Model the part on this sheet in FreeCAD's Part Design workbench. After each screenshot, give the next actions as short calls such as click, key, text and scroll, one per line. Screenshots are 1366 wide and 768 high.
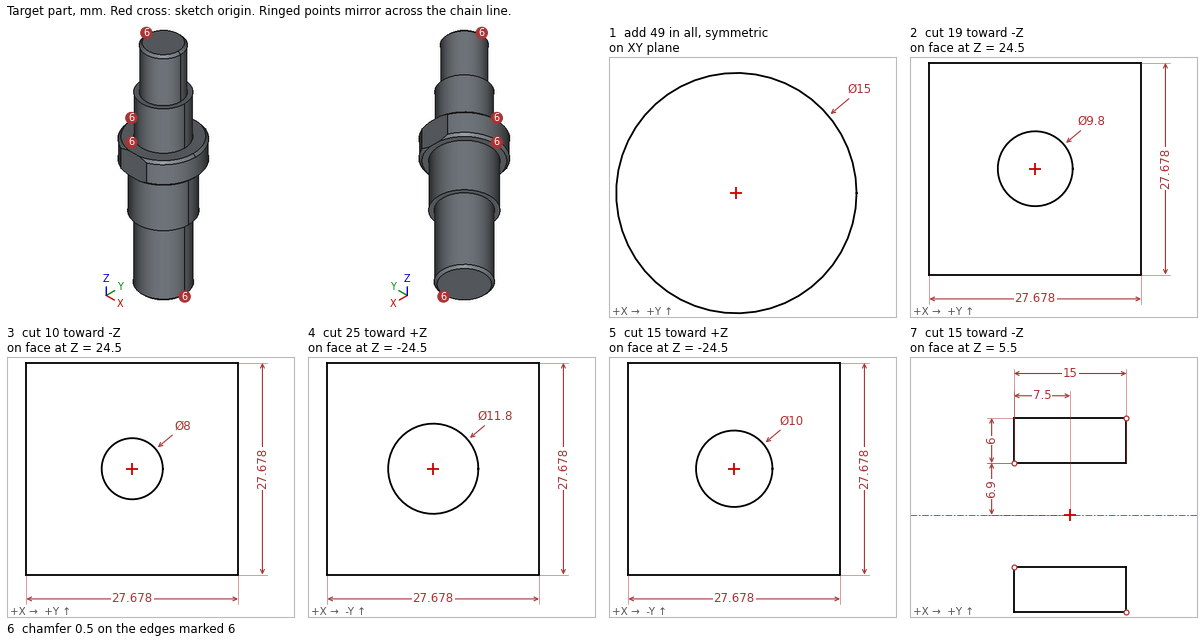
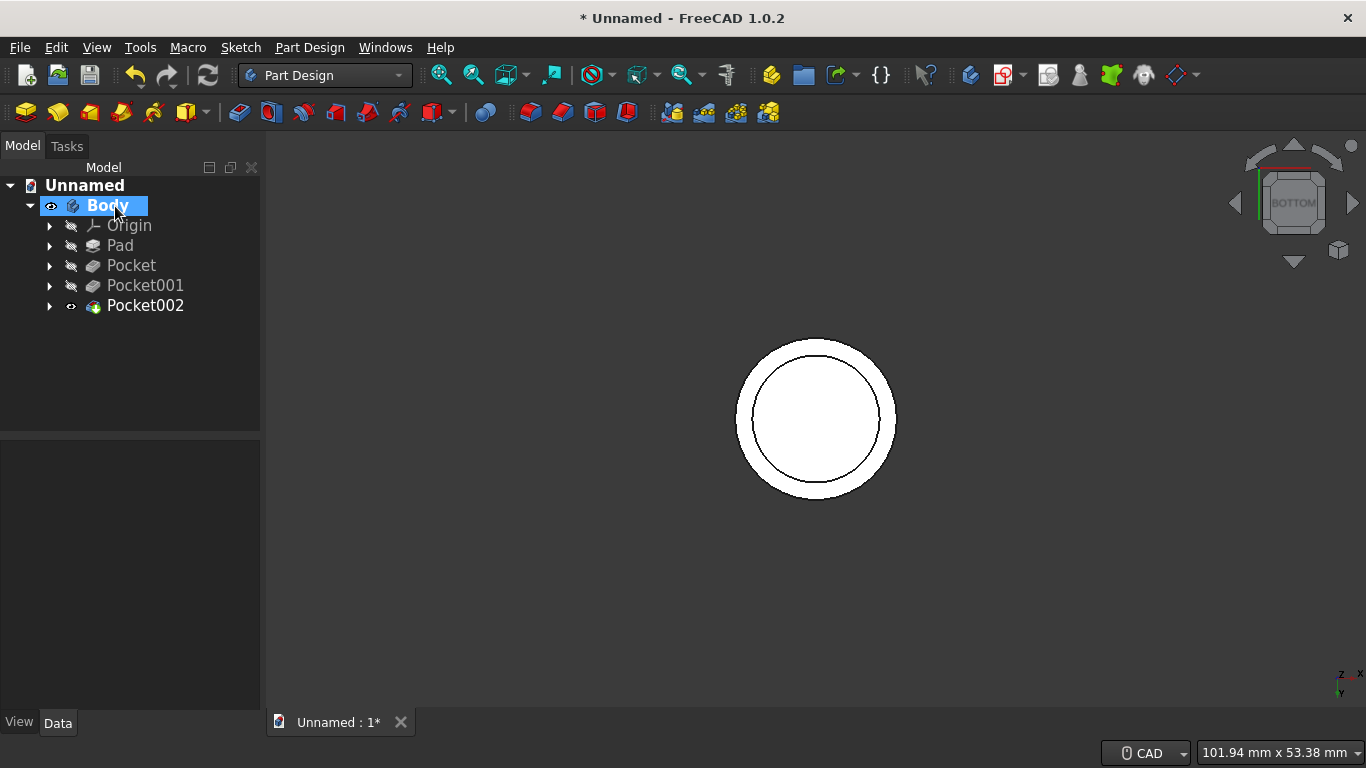
click(442, 76)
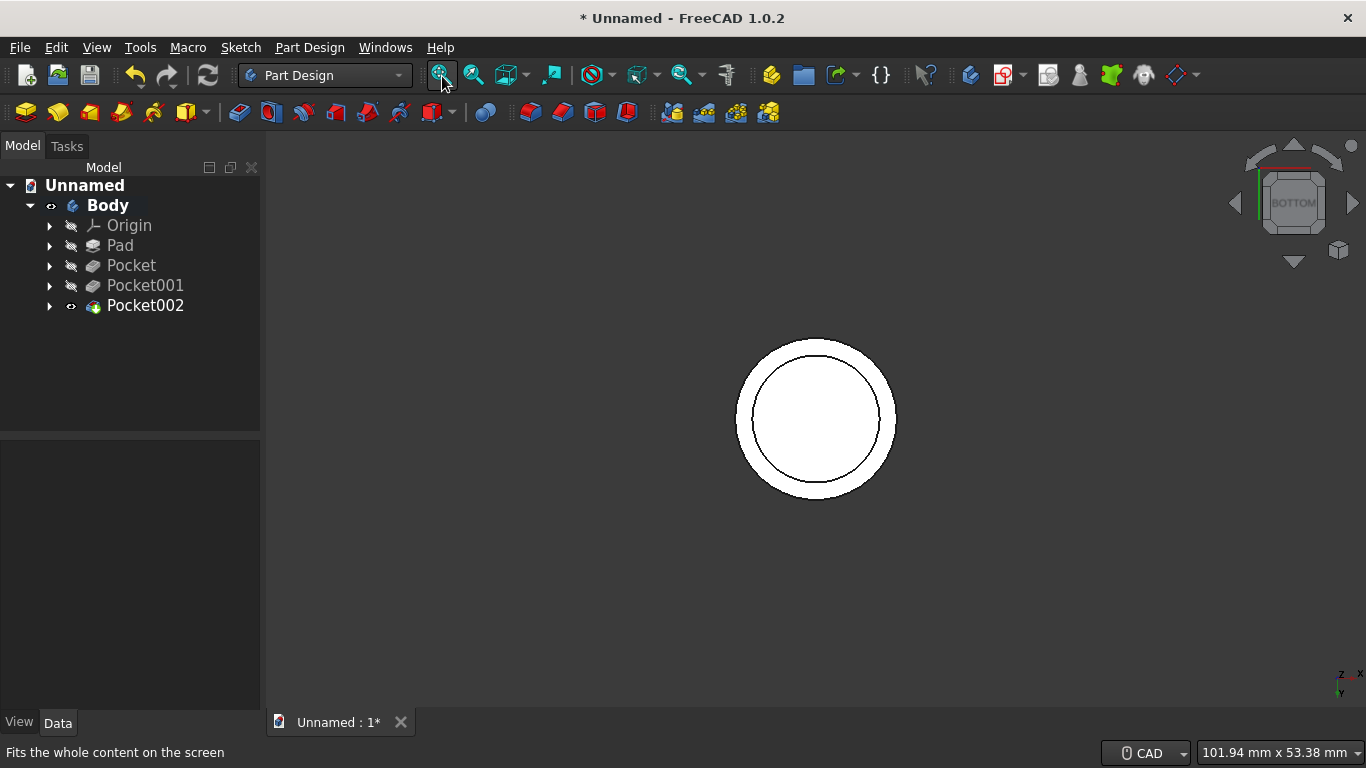
click(816, 418)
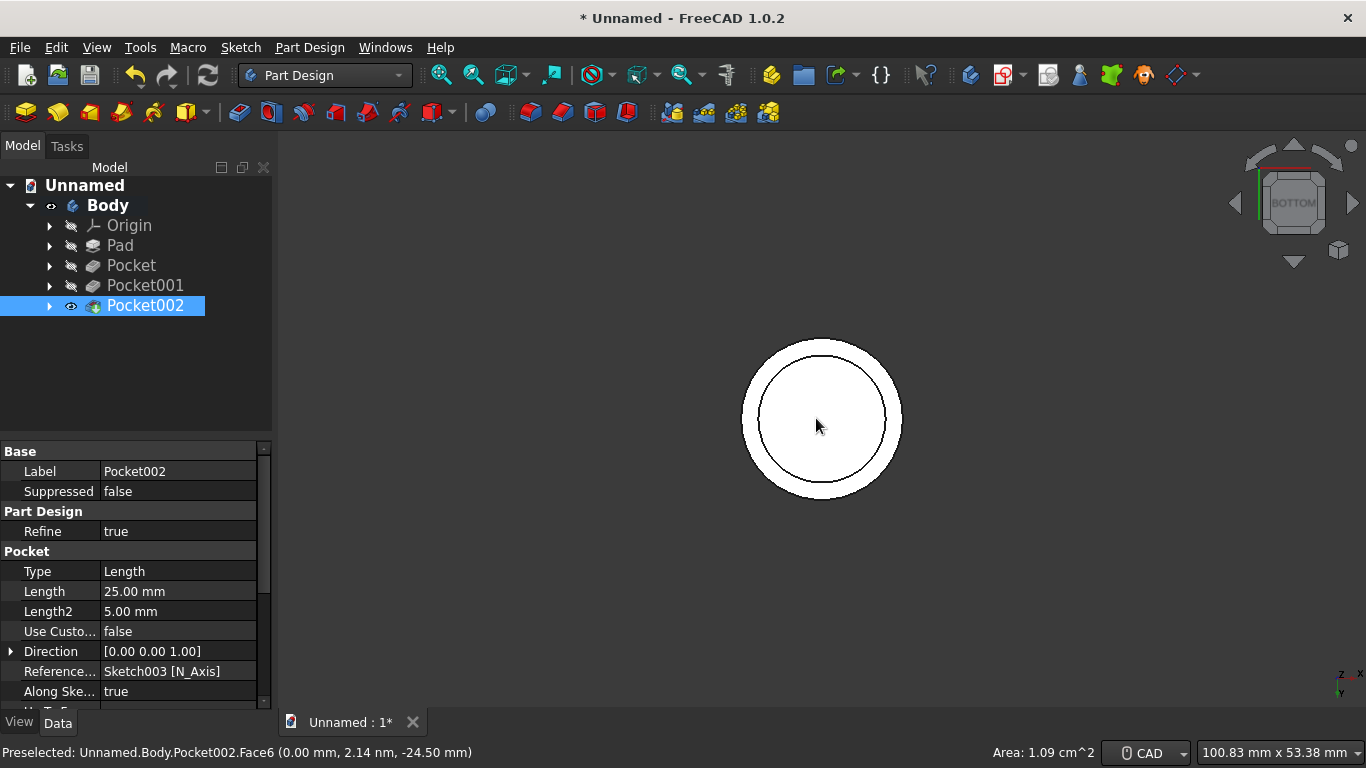
click(1004, 76)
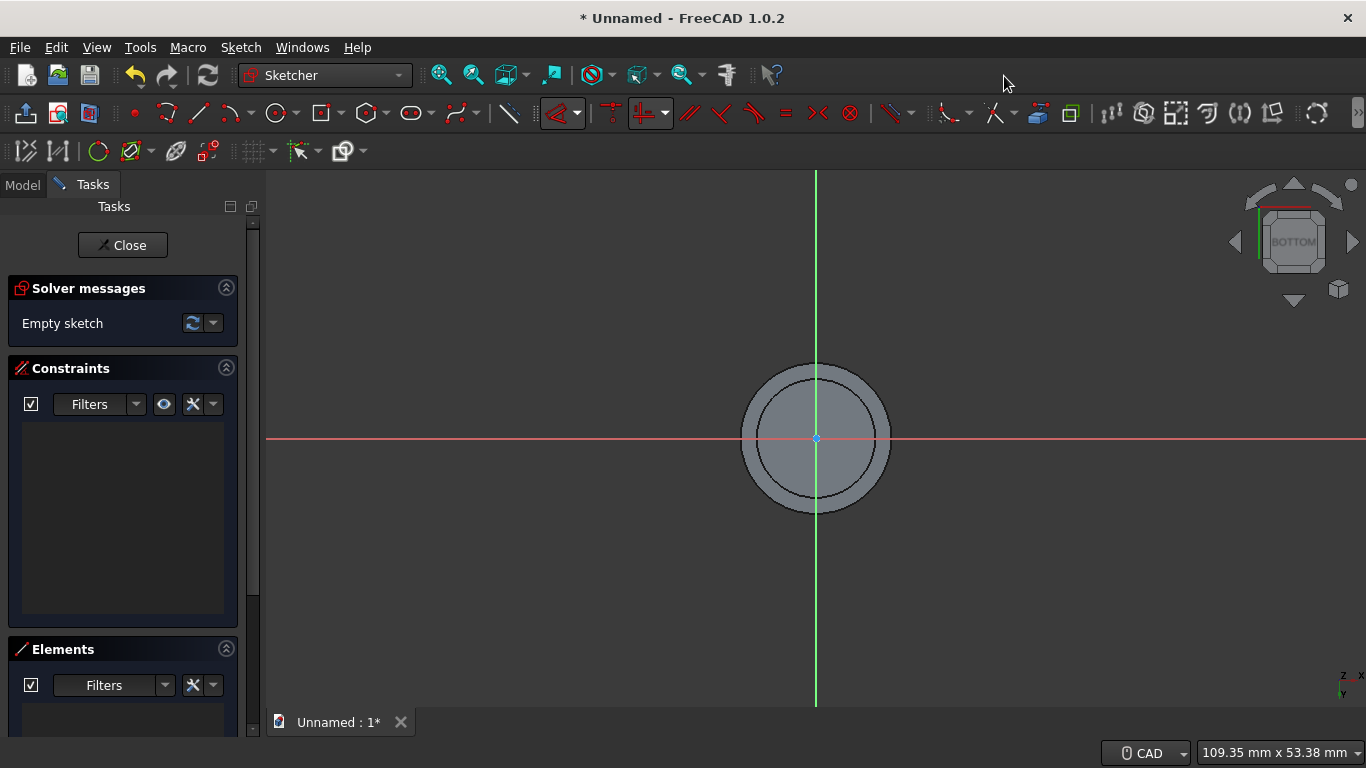
click(322, 114)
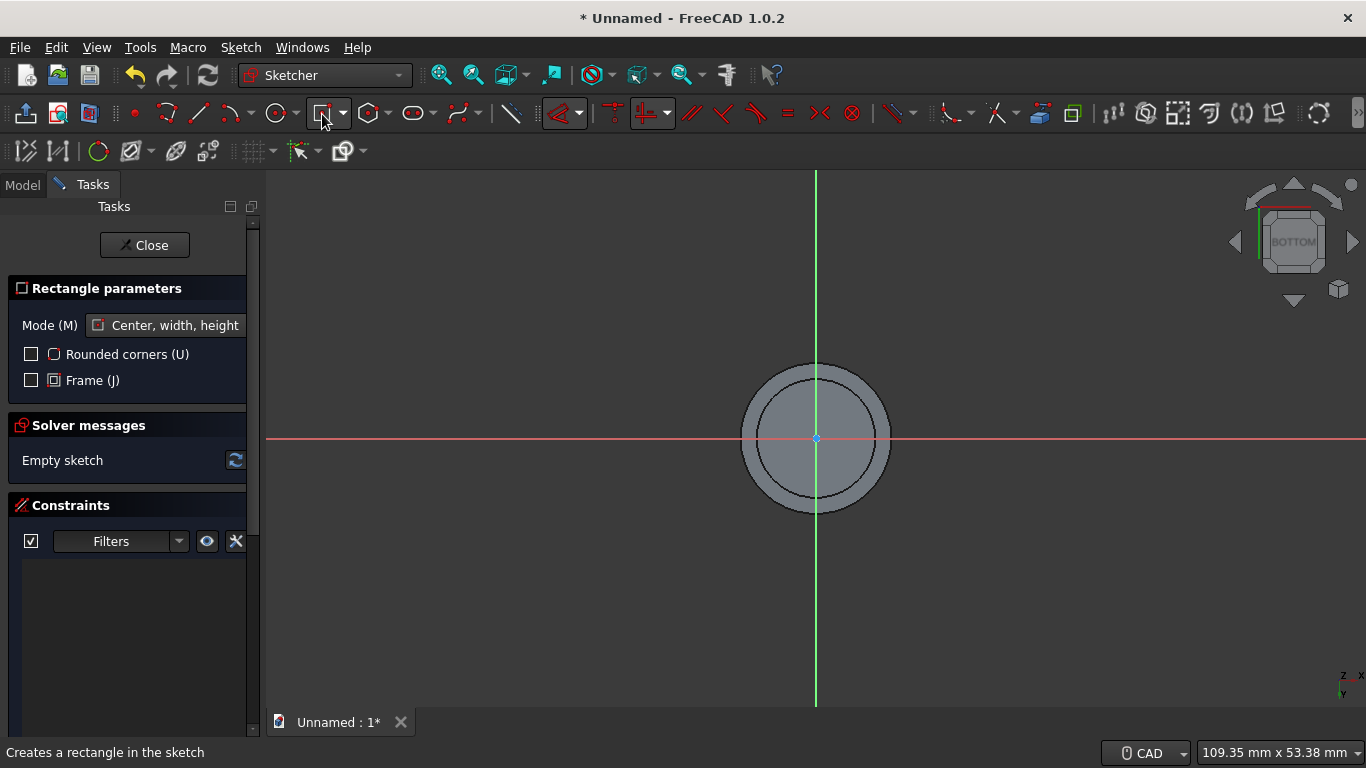
click(816, 438)
click(955, 299)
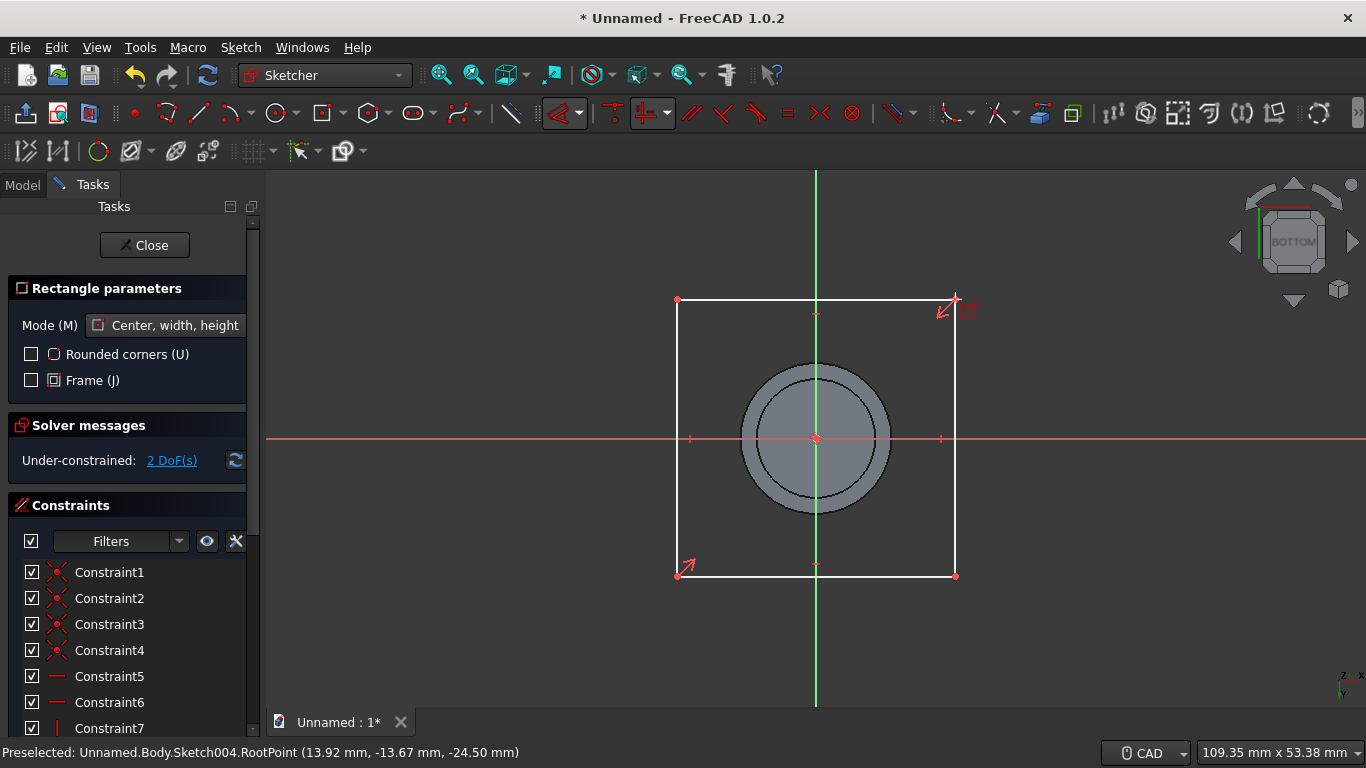
click(276, 114)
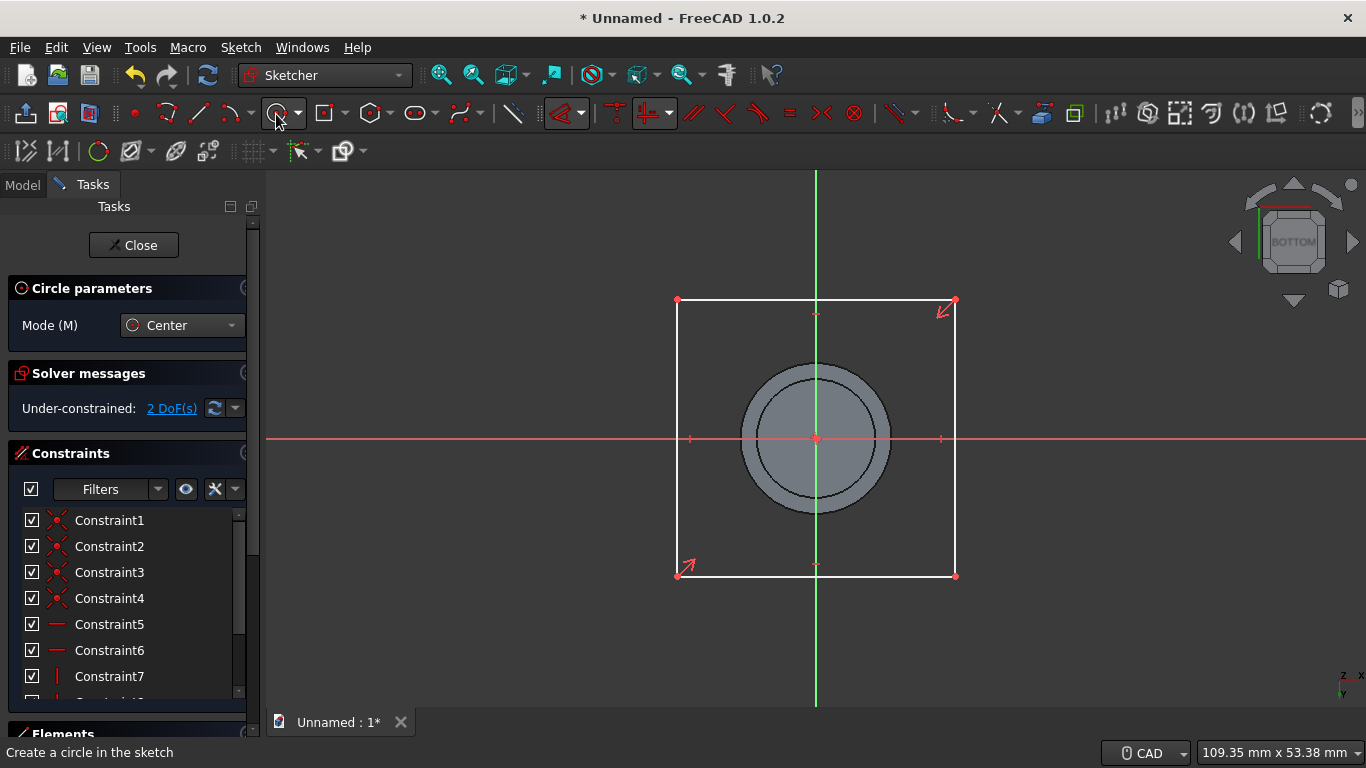
click(816, 438)
click(852, 403)
key(Escape)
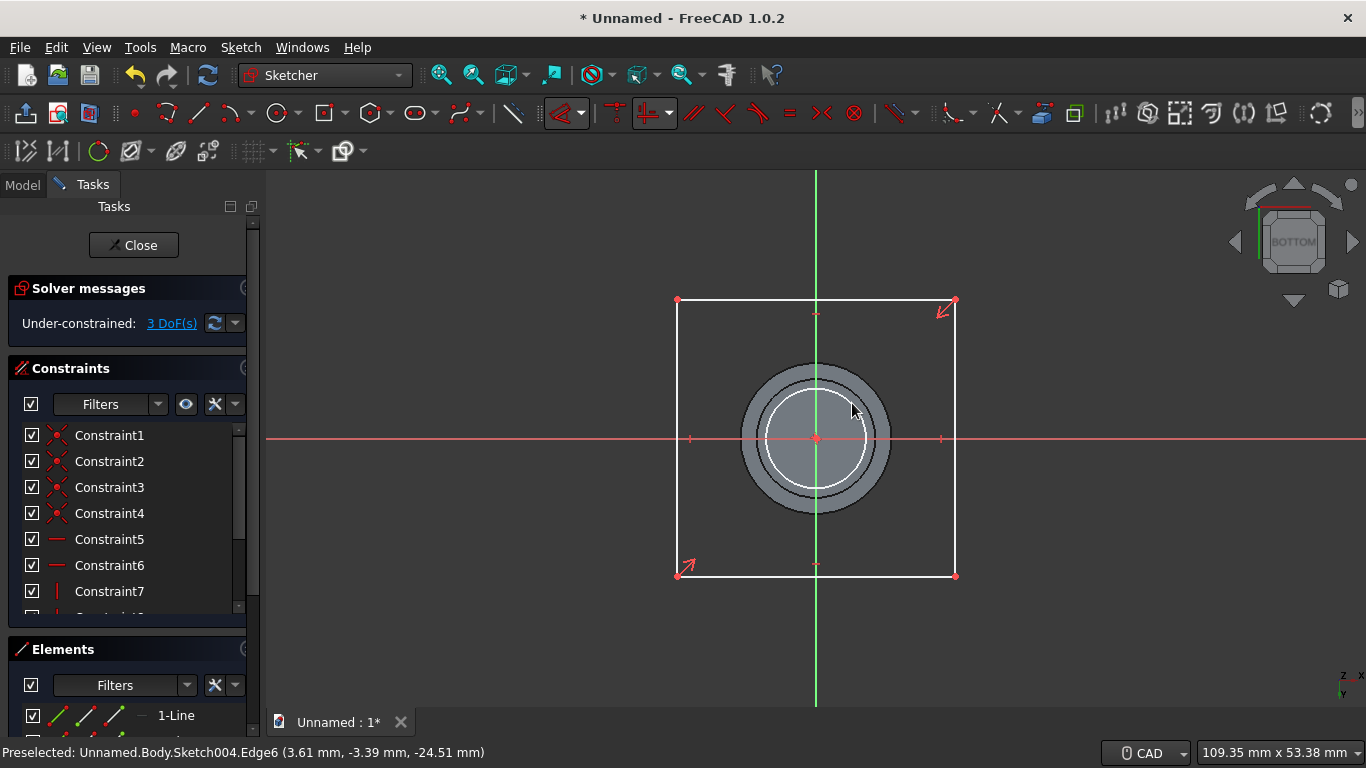
click(851, 403)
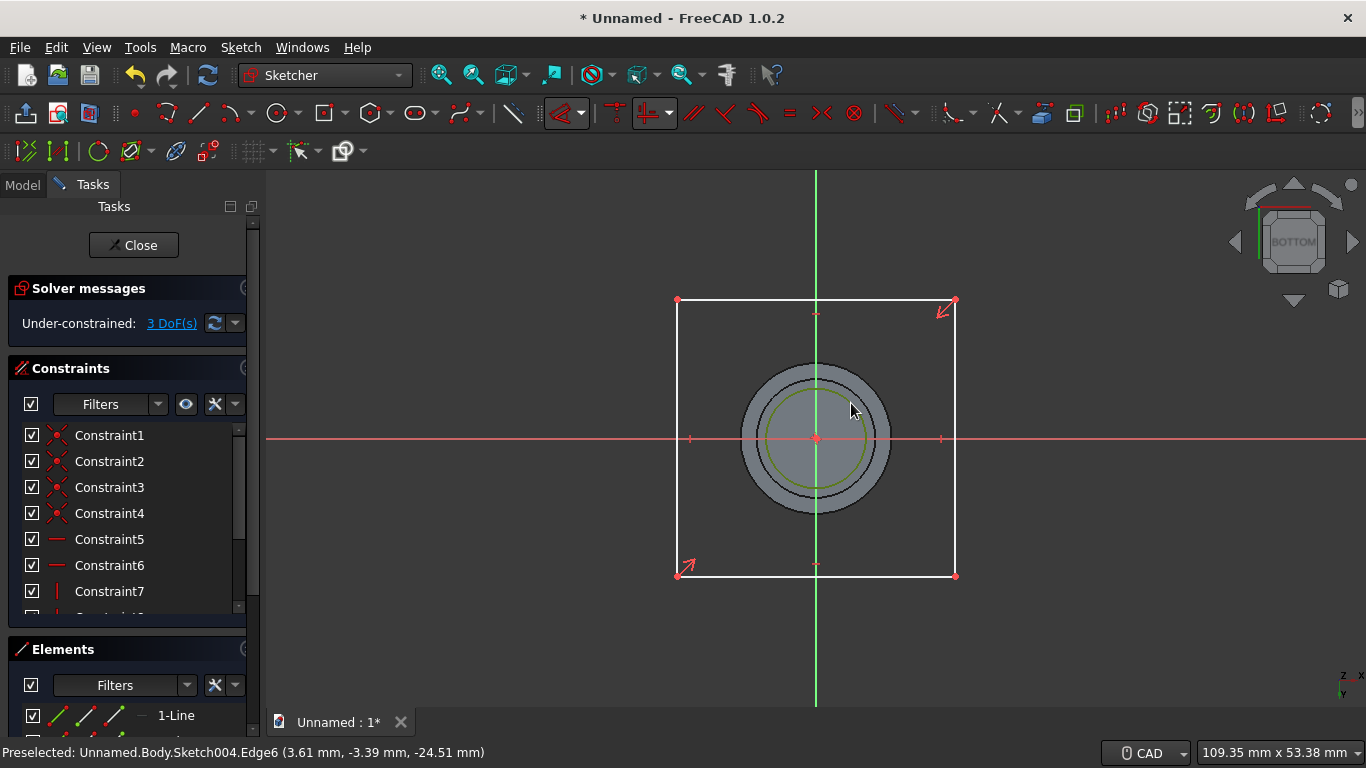
key(k)
key(o)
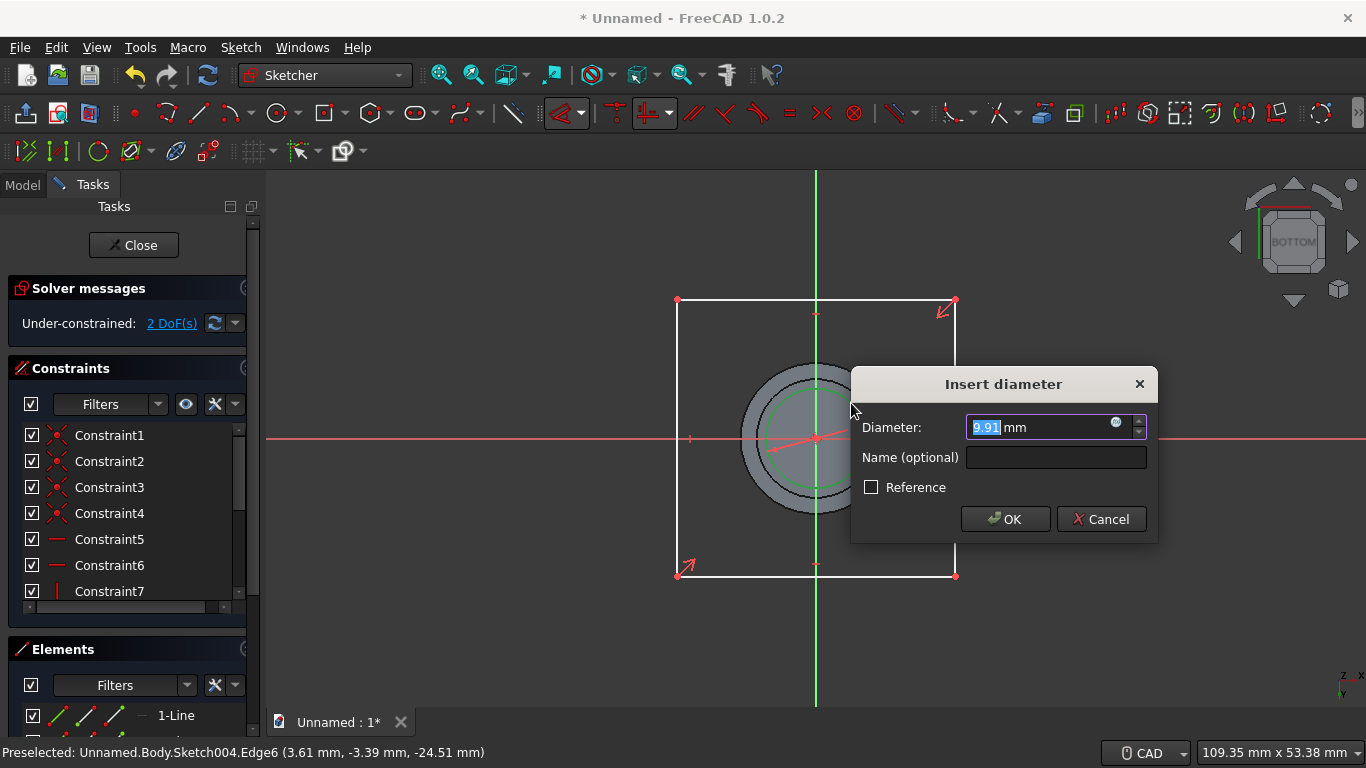
text(10)
key(Return)